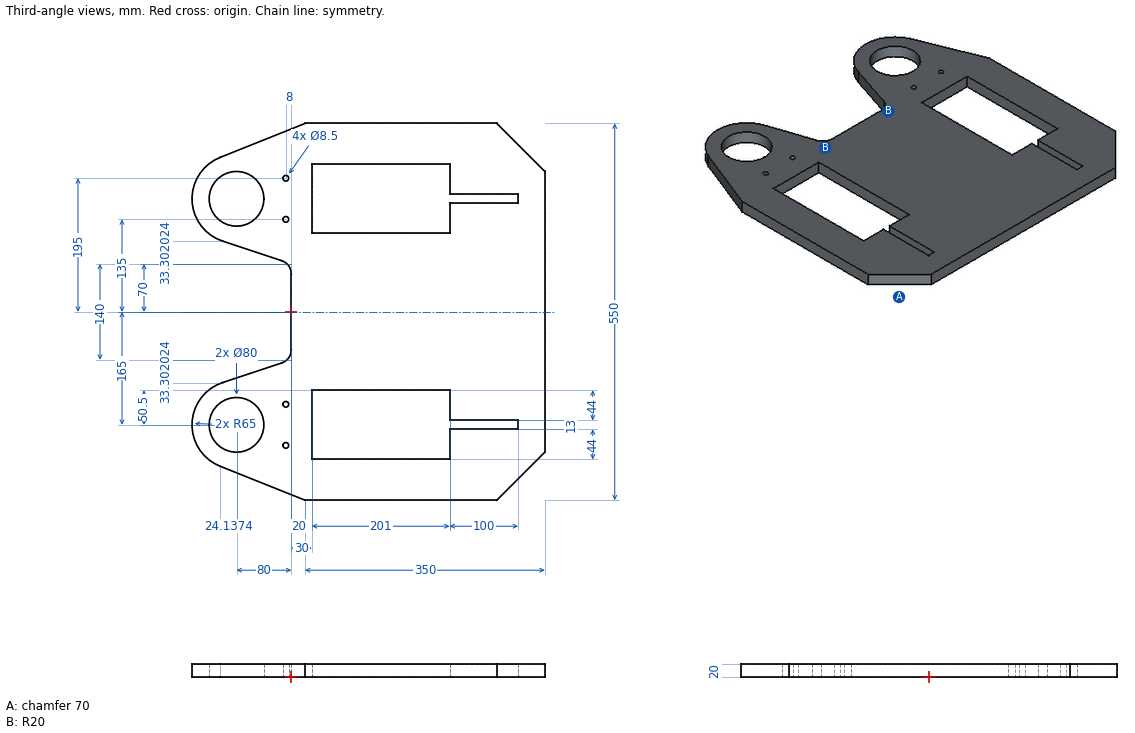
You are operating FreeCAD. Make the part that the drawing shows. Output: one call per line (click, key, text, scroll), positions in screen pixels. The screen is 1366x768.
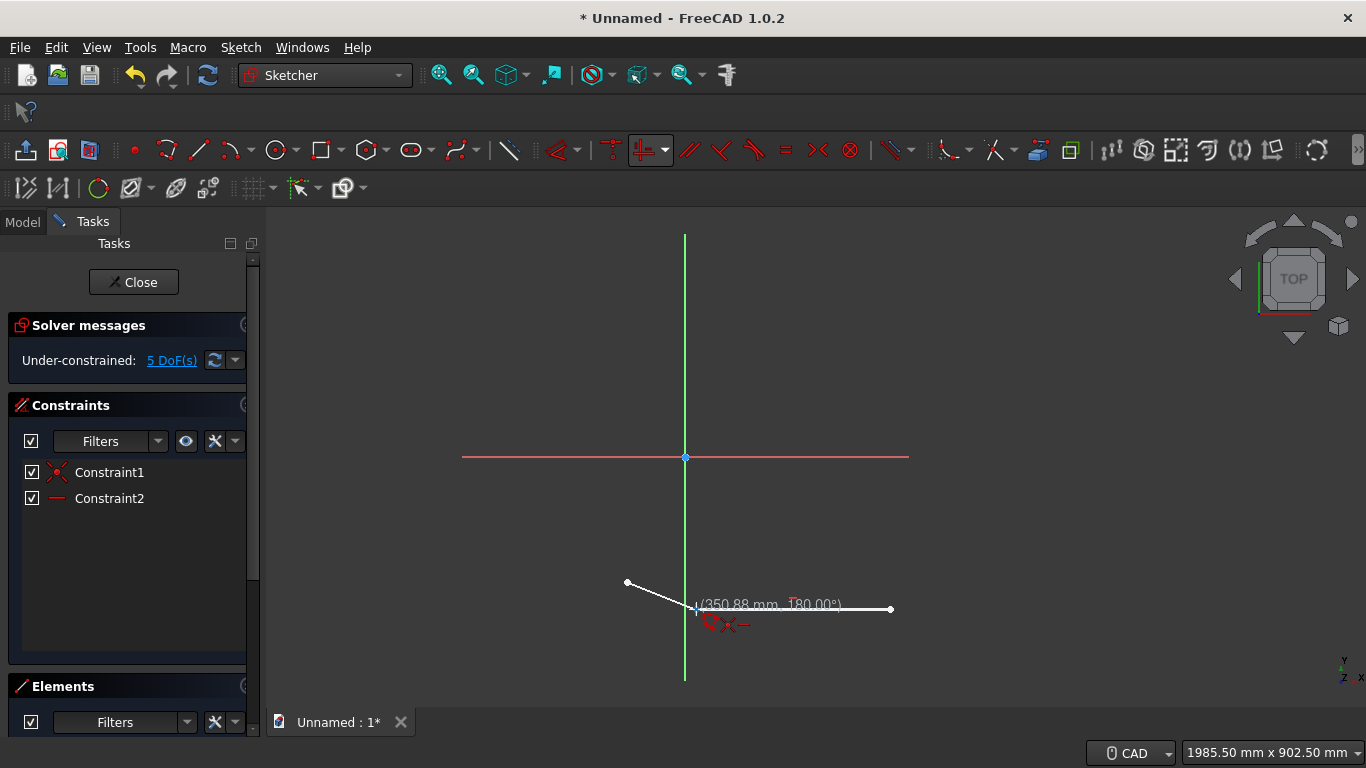
click(891, 305)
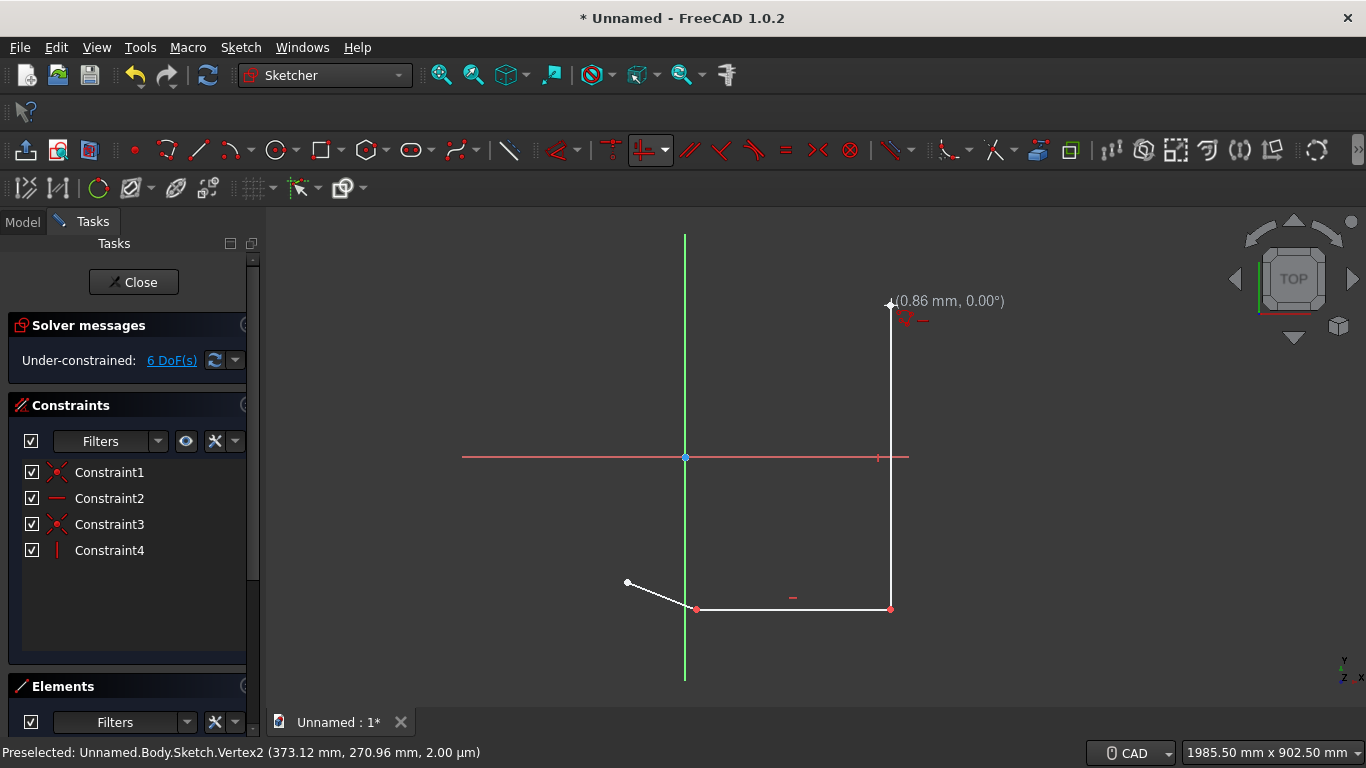
scroll(696, 305, up, 2)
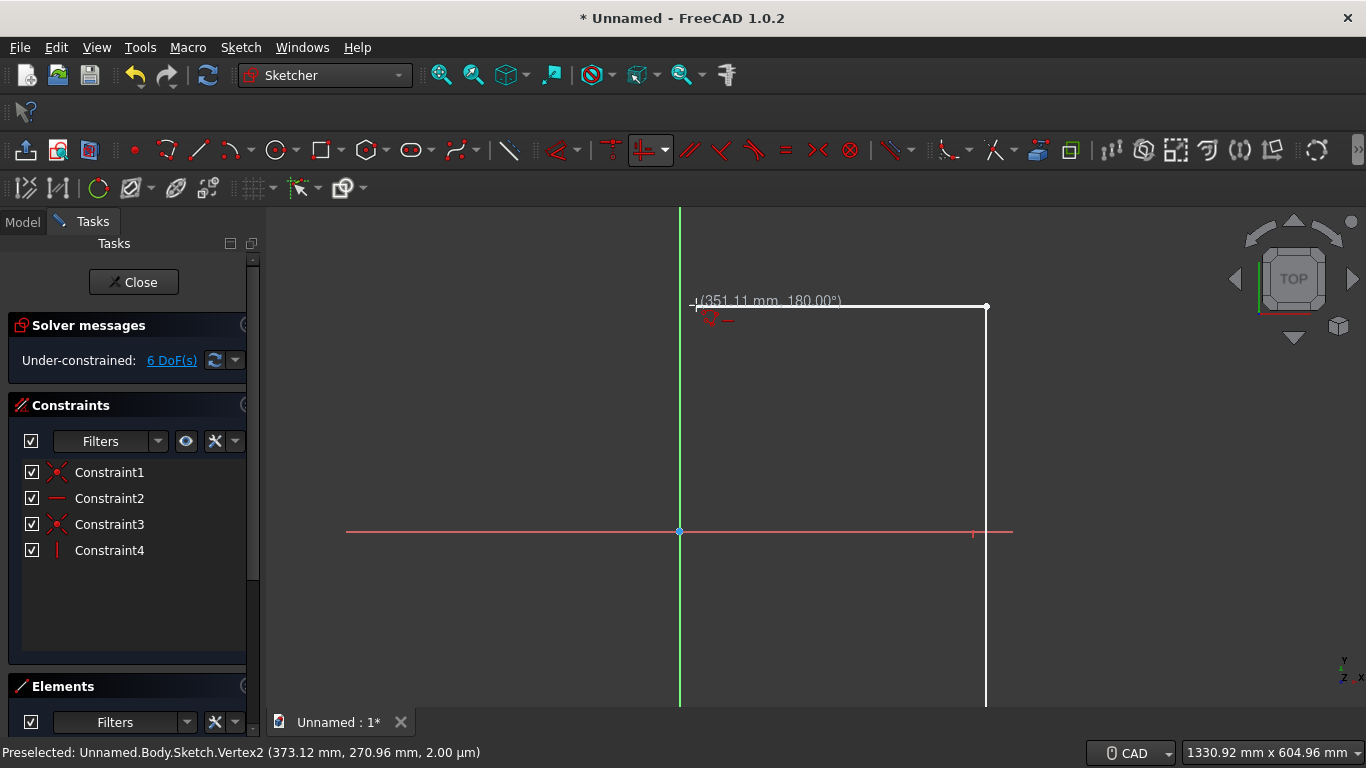
click(696, 305)
click(594, 346)
right_click(594, 346)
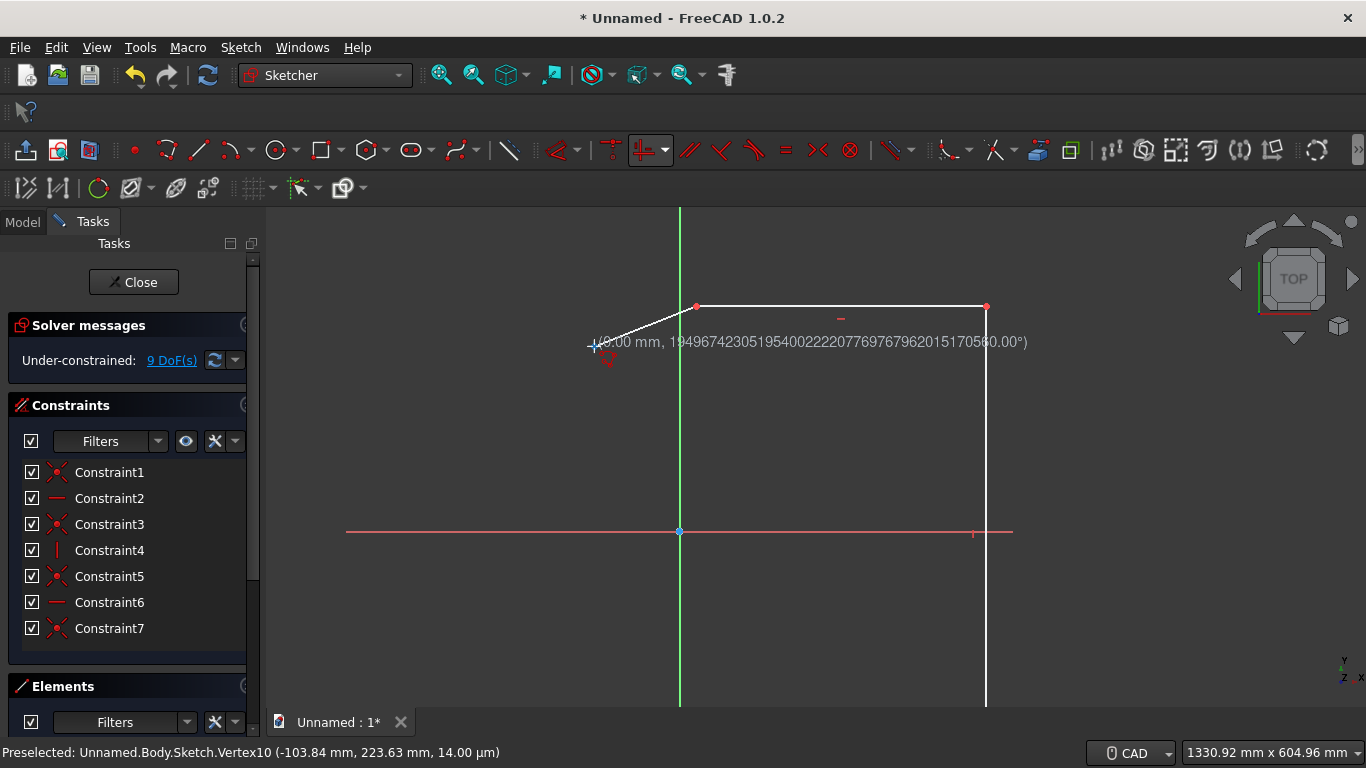
click(597, 446)
click(680, 474)
click(689, 590)
click(597, 617)
right_click(597, 617)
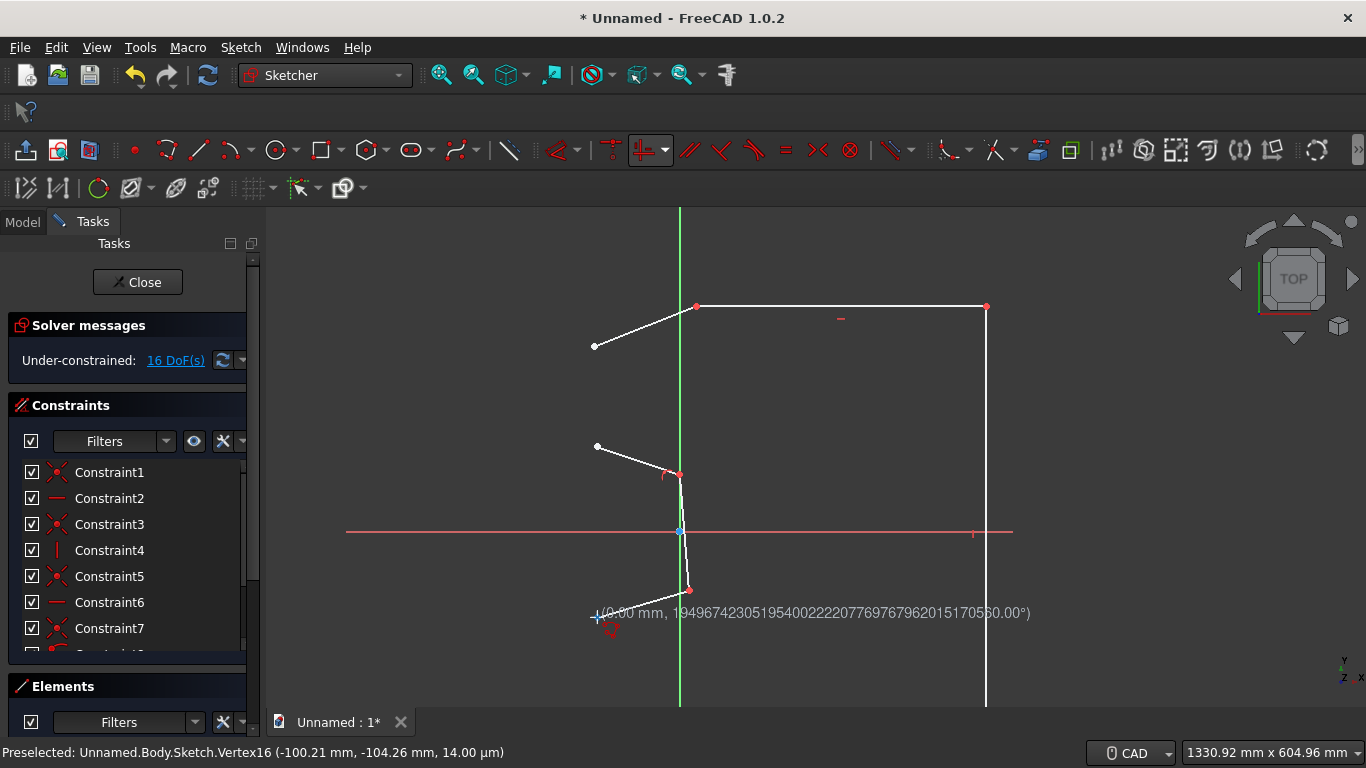
key(g)
key(3)
key(a)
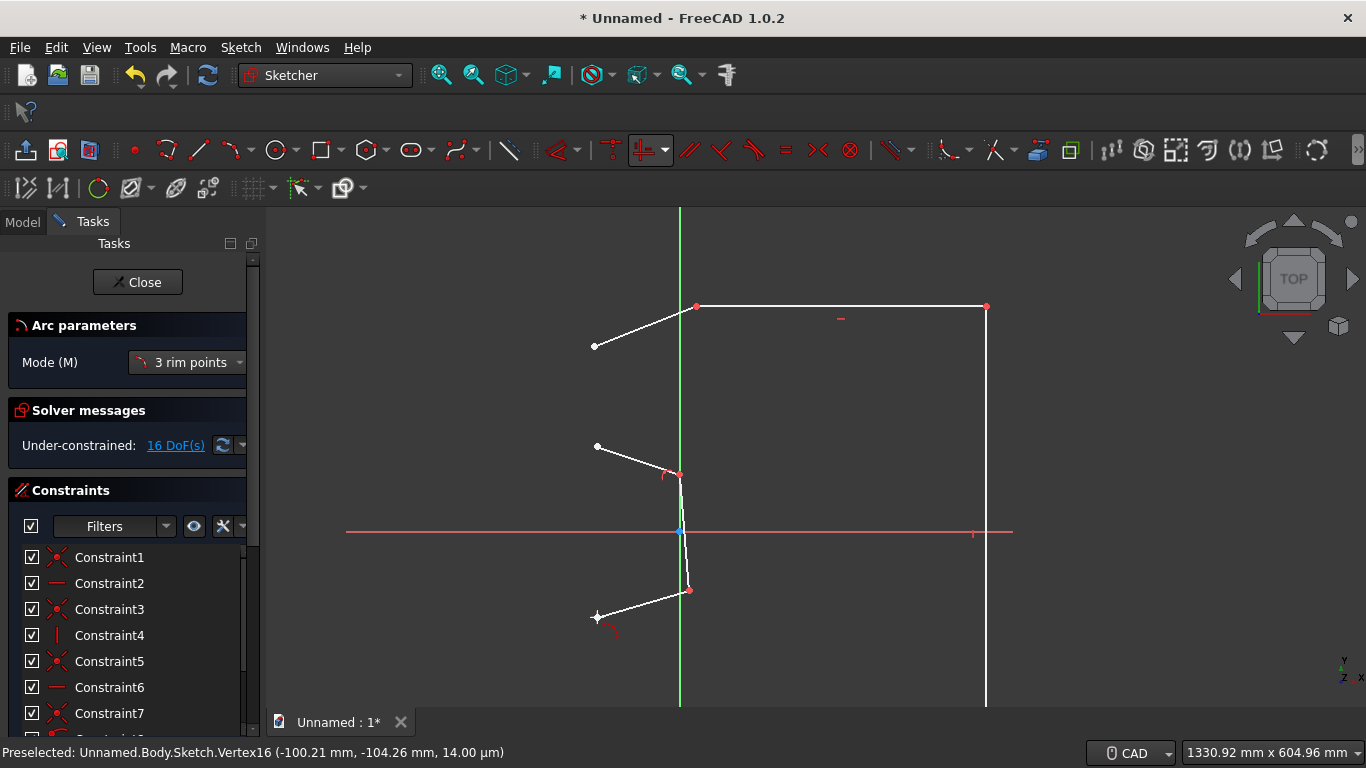
click(594, 347)
click(597, 447)
click(560, 397)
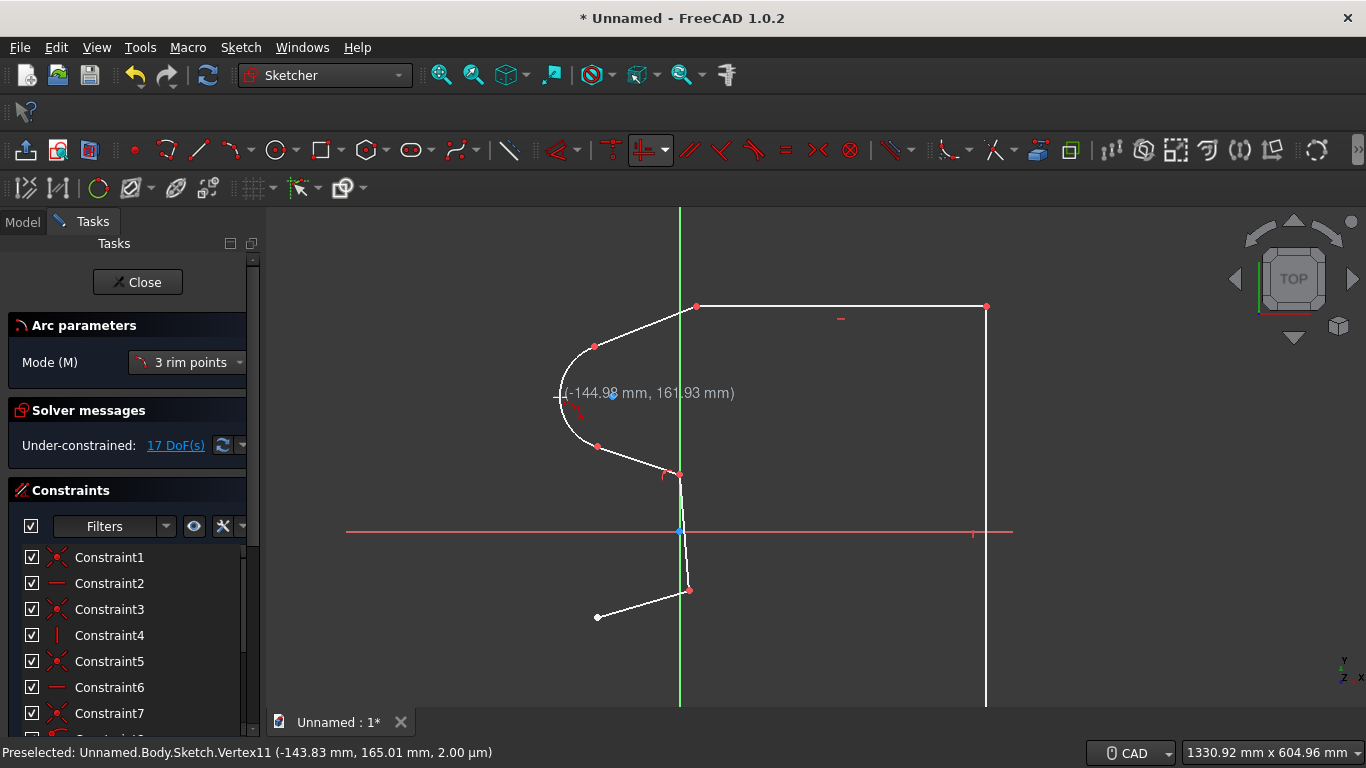
click(597, 618)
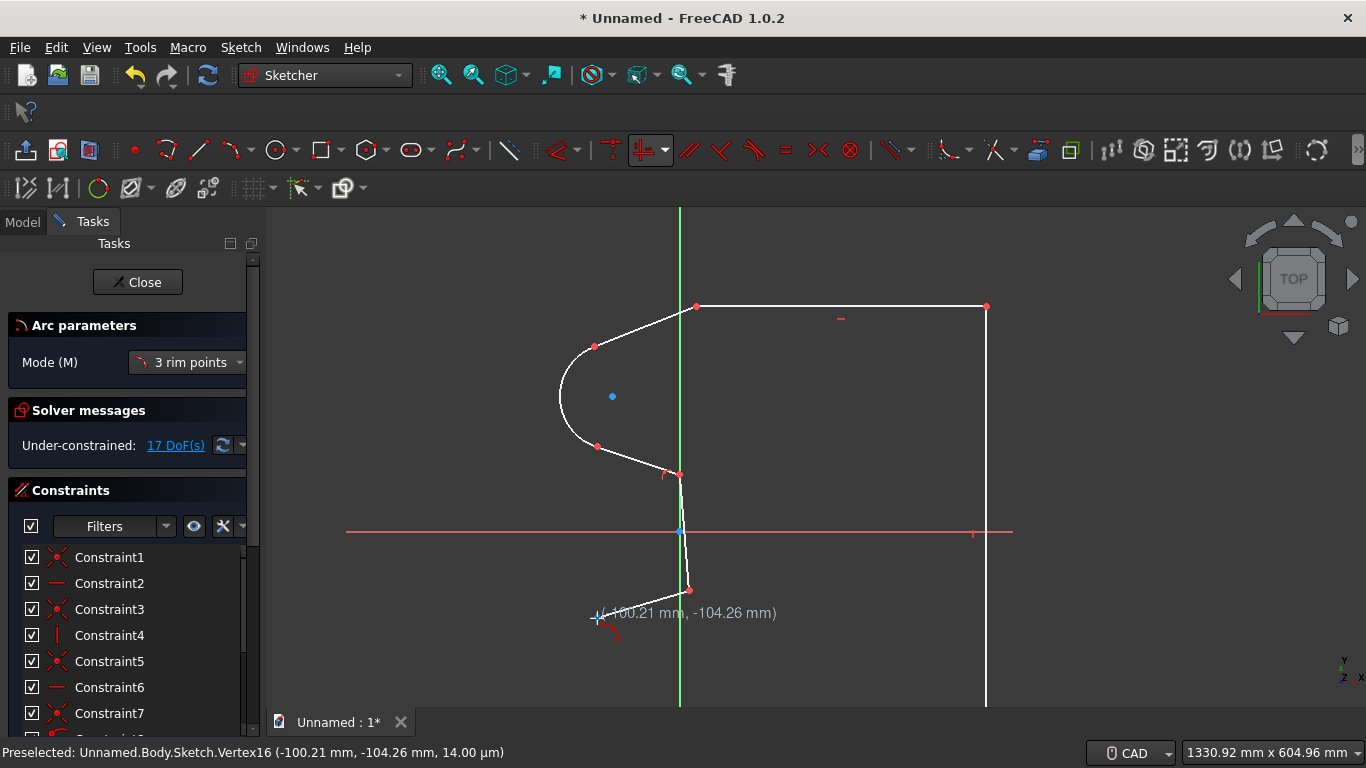
scroll(696, 305, down, 2)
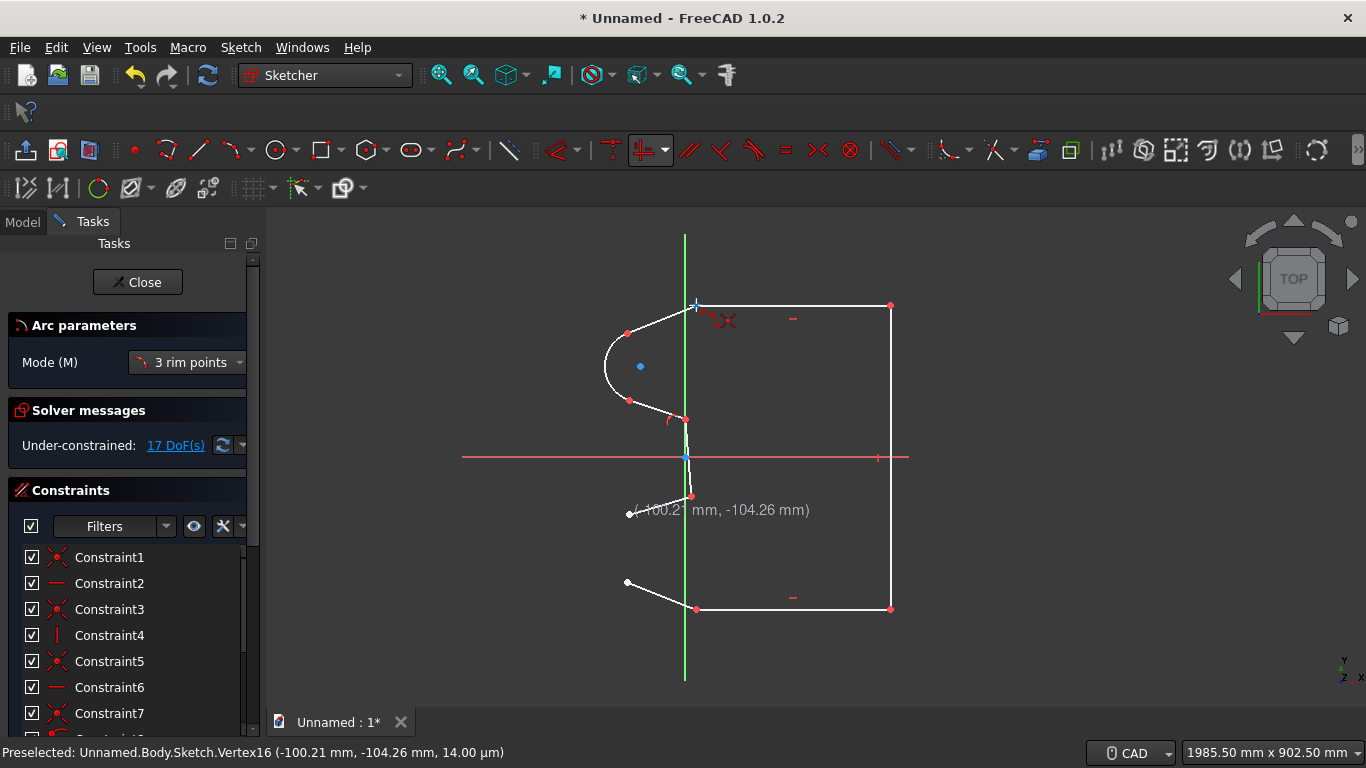
click(628, 583)
click(605, 547)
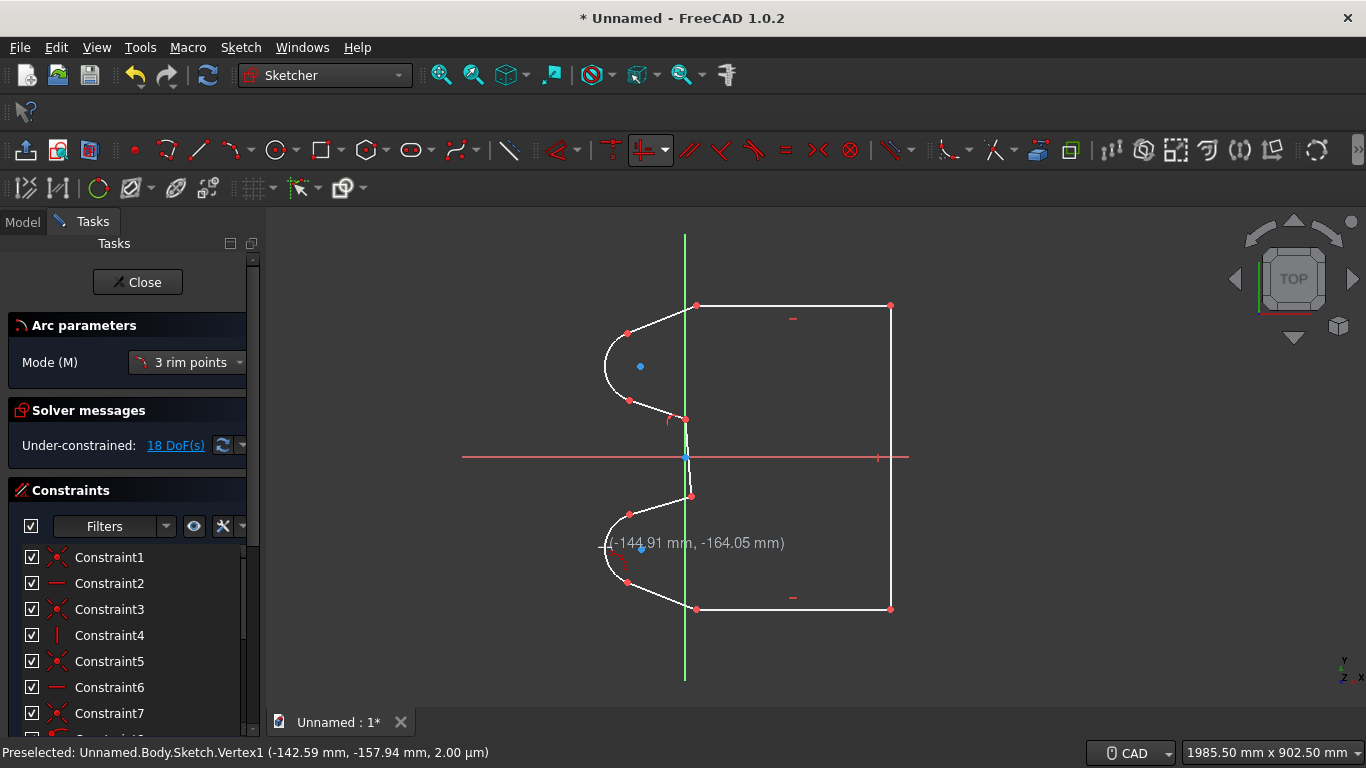
click(168, 150)